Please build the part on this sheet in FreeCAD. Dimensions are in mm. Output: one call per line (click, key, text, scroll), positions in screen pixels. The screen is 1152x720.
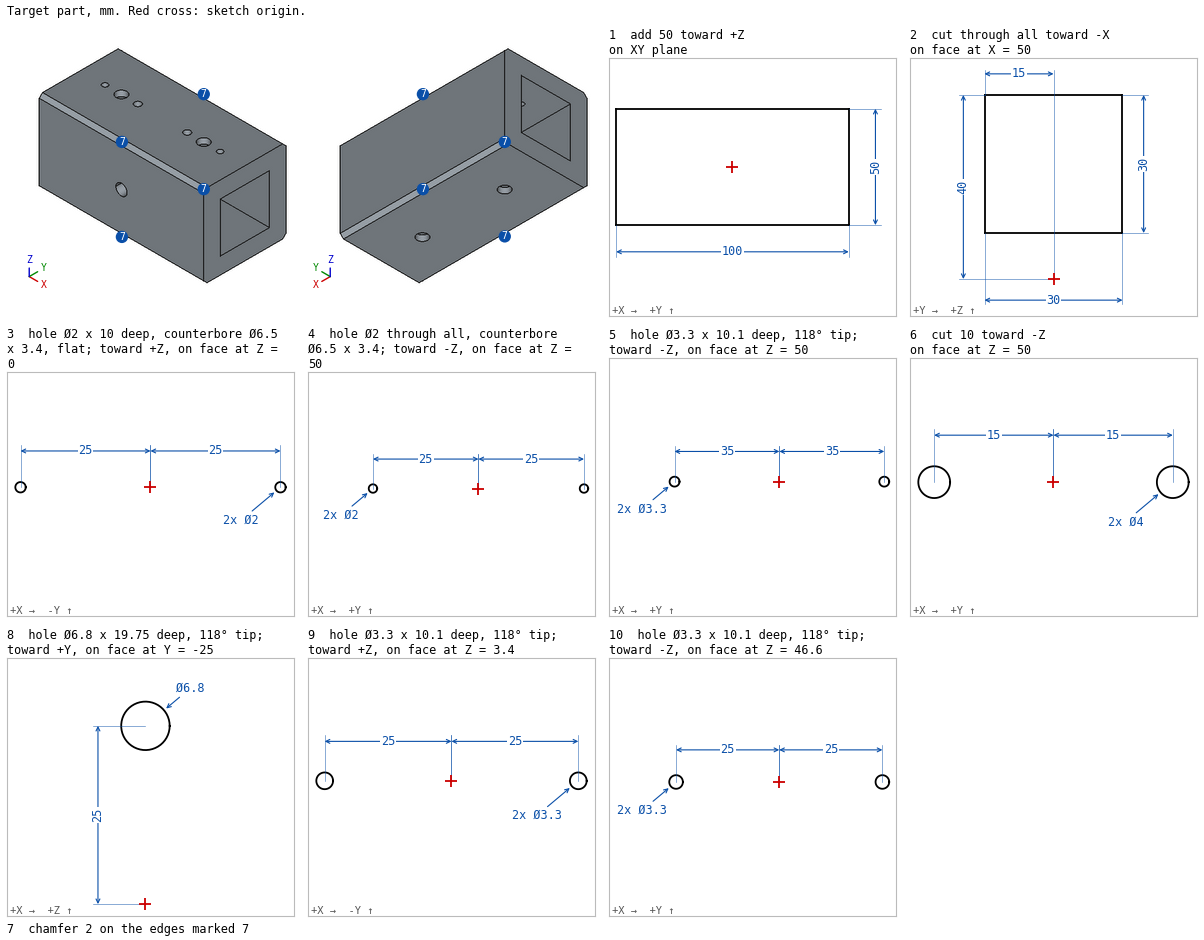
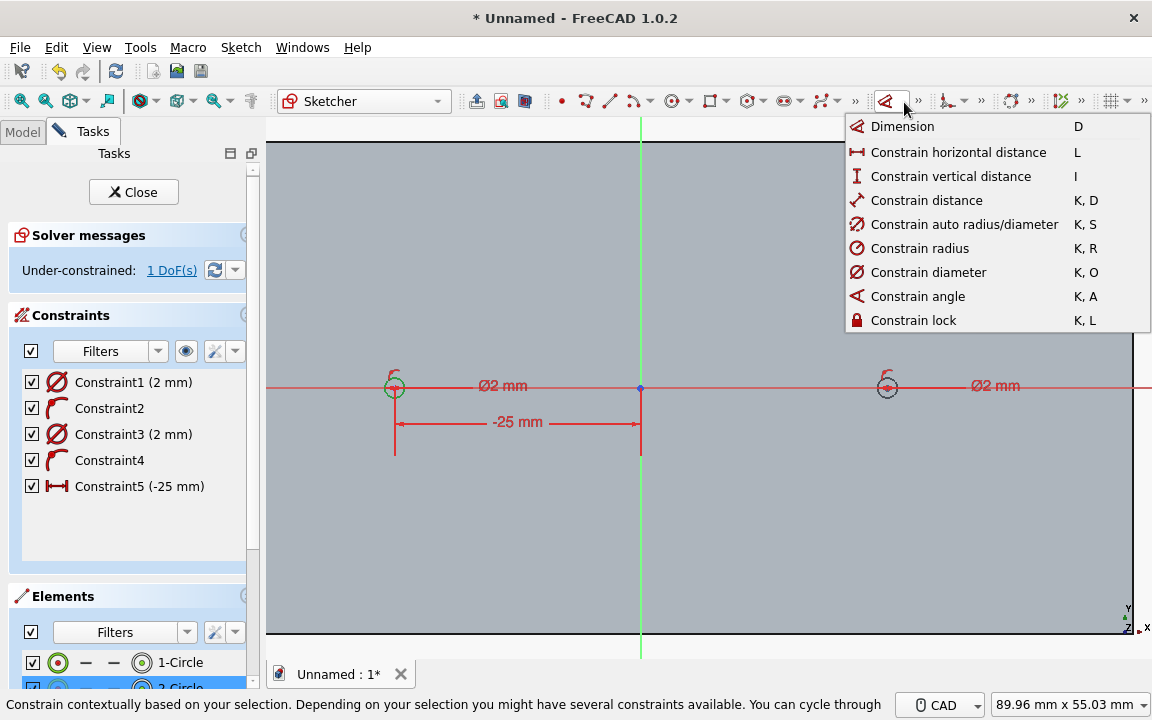
click(998, 152)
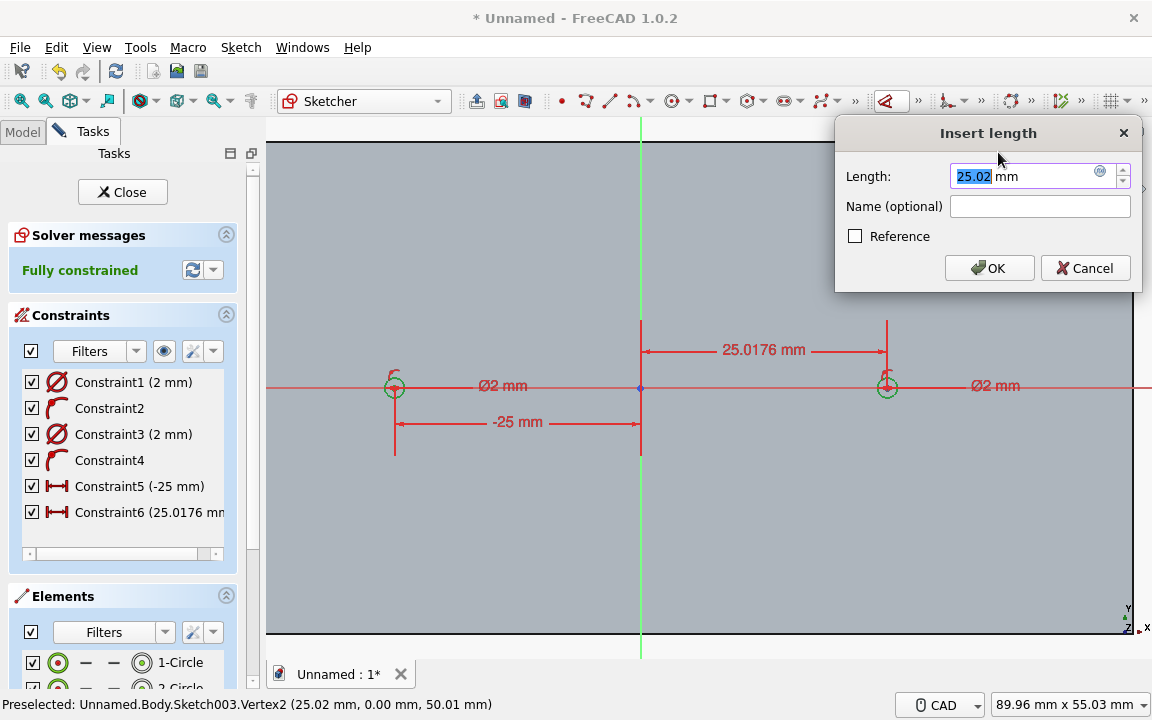
text(25)
key(Return)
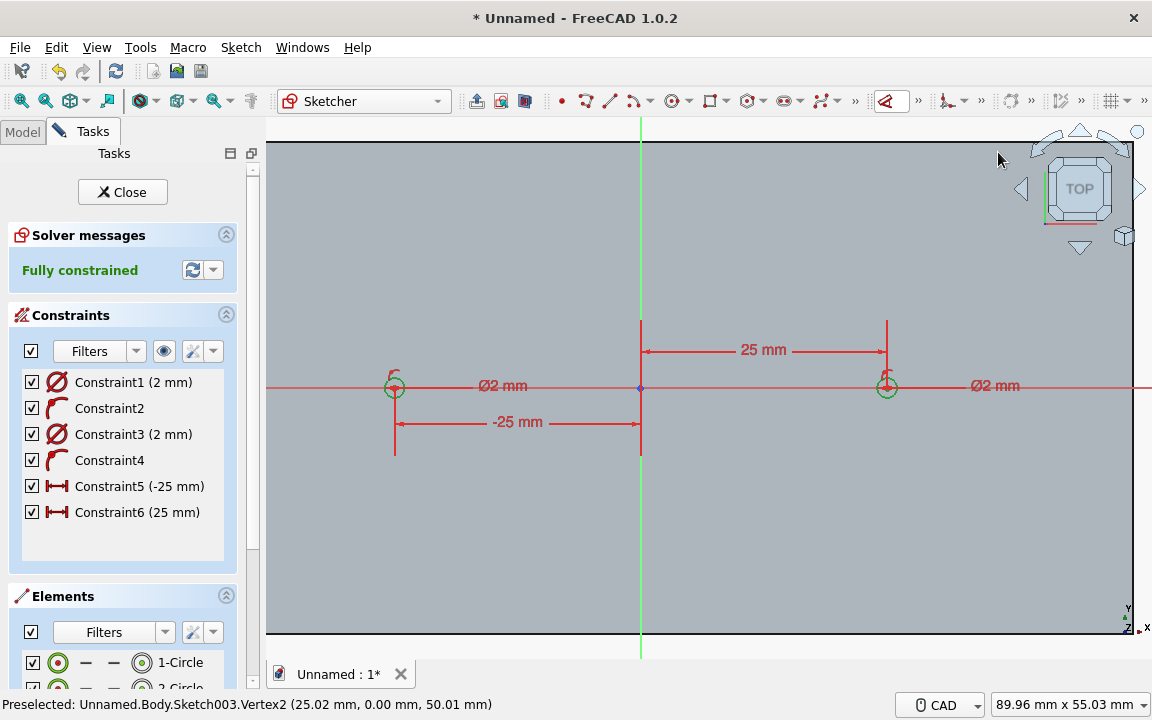
click(123, 192)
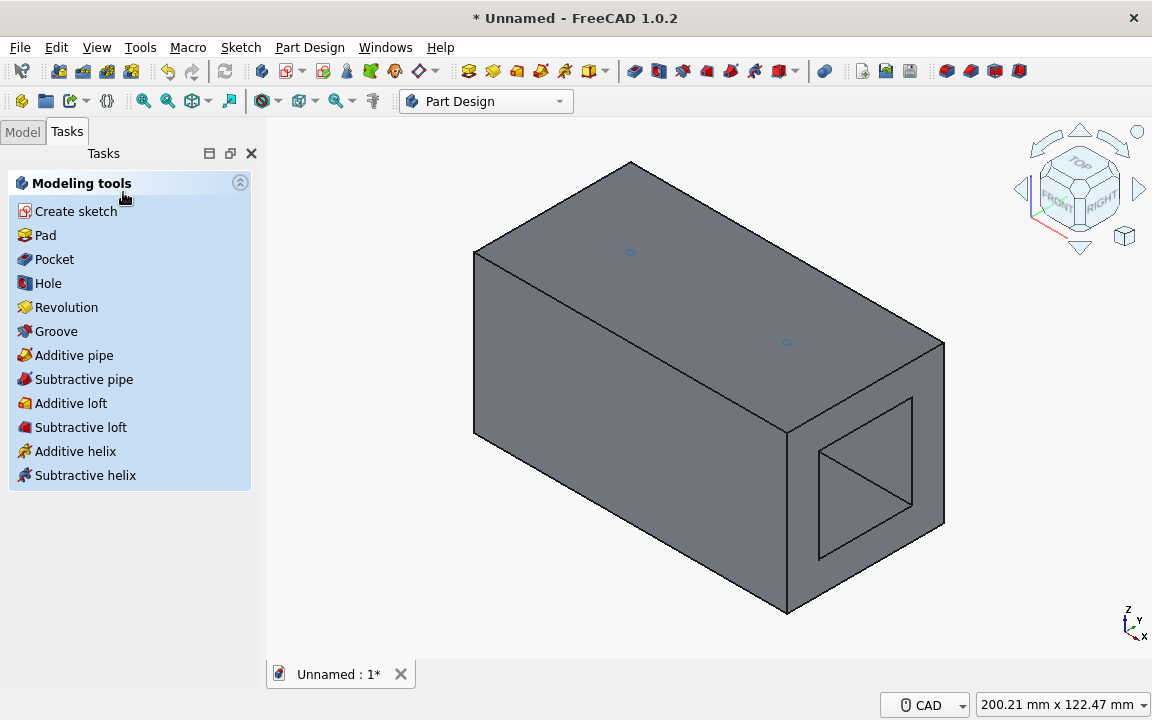
click(660, 72)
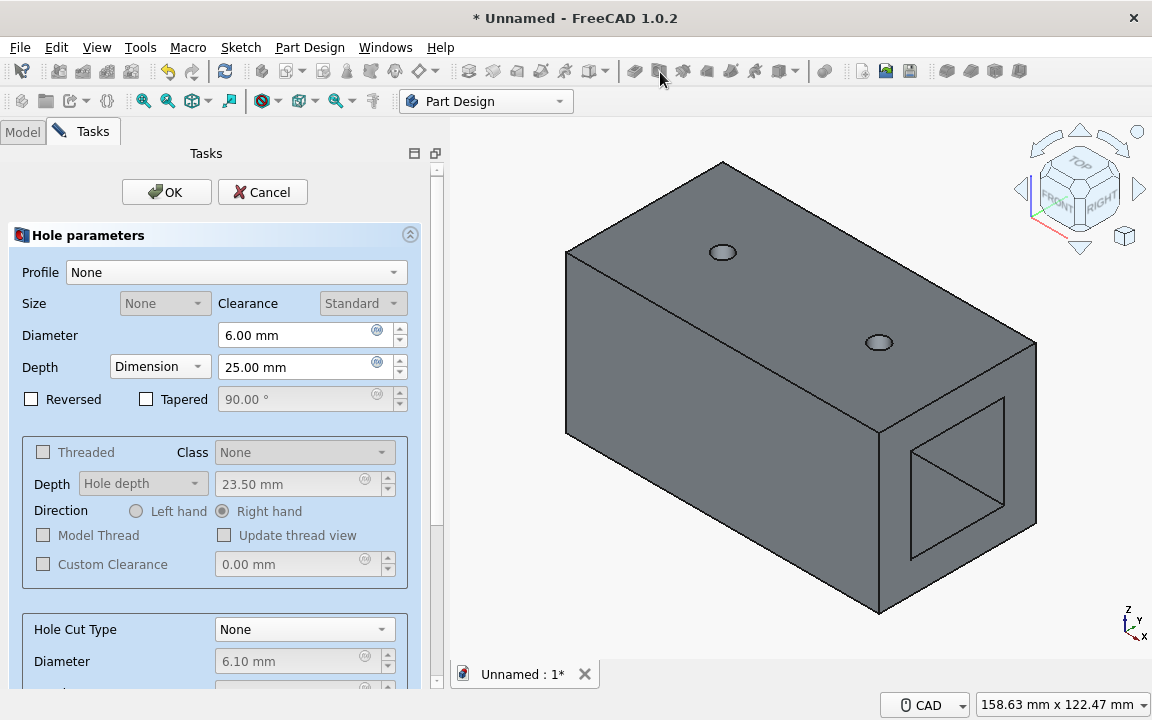
triple_click(305, 335)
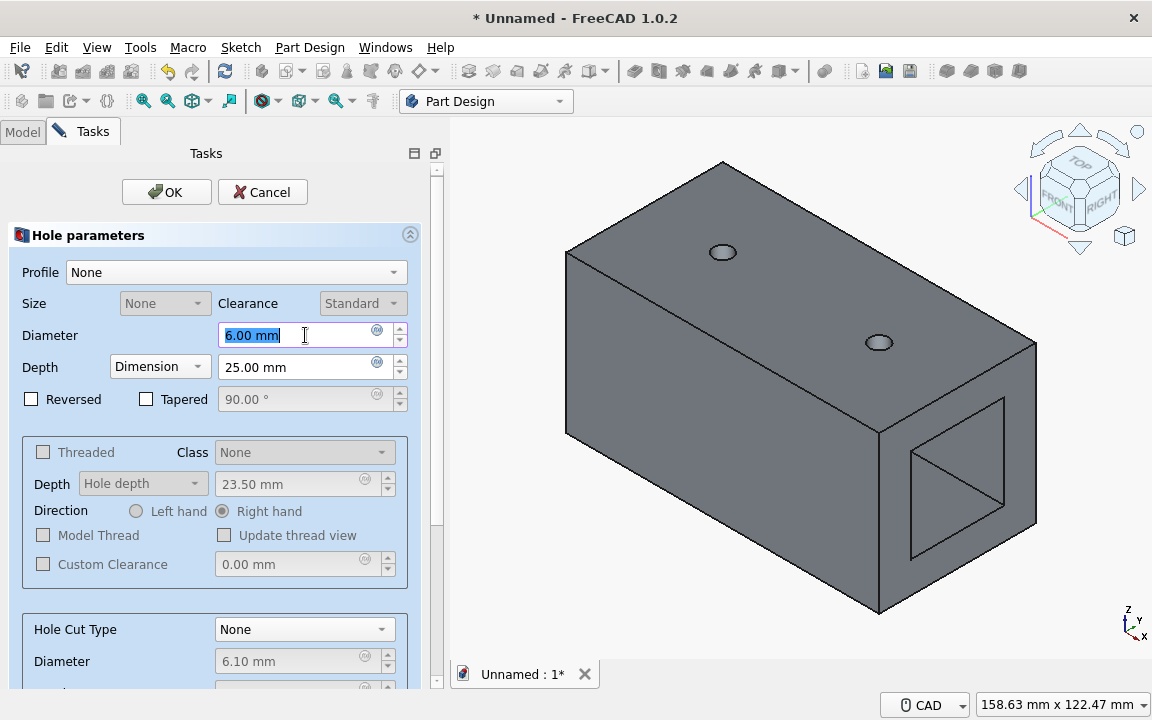
text(2)
key(Tab)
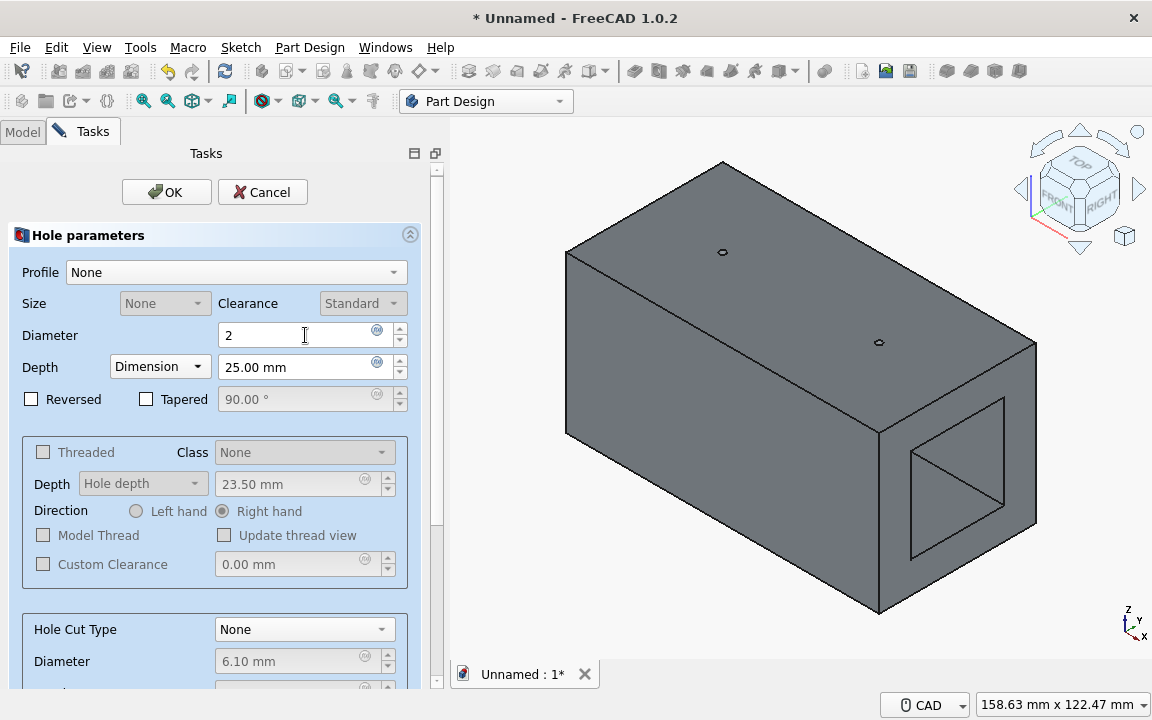
click(161, 366)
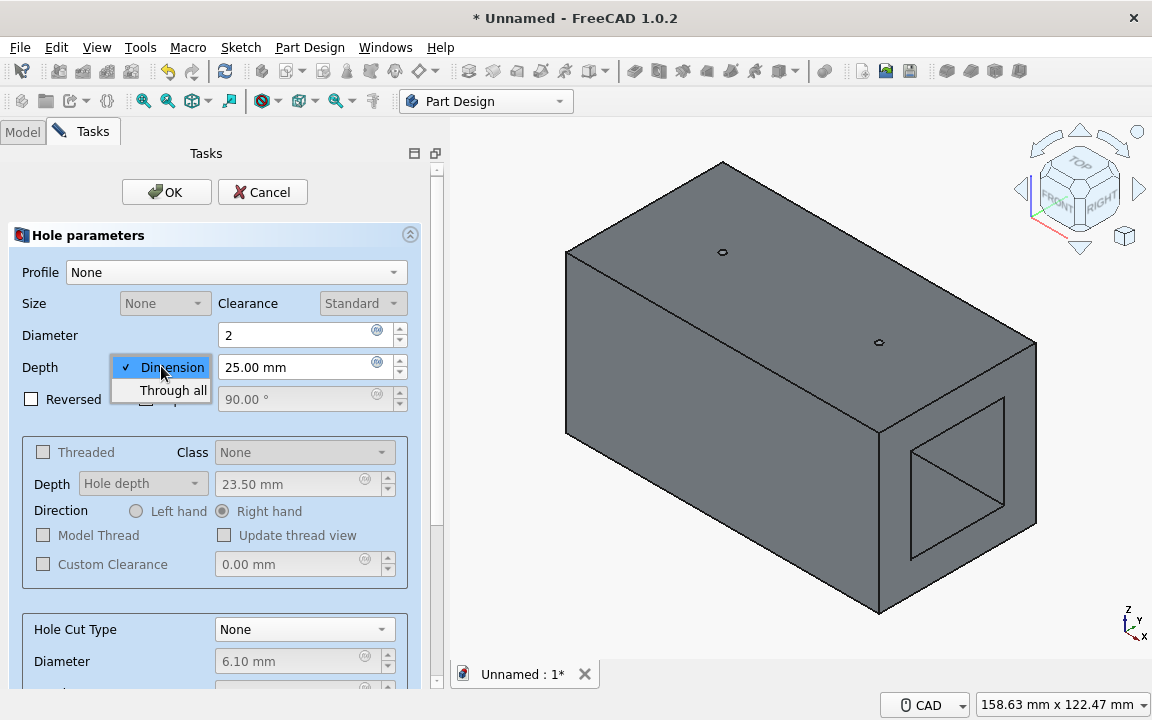
click(160, 390)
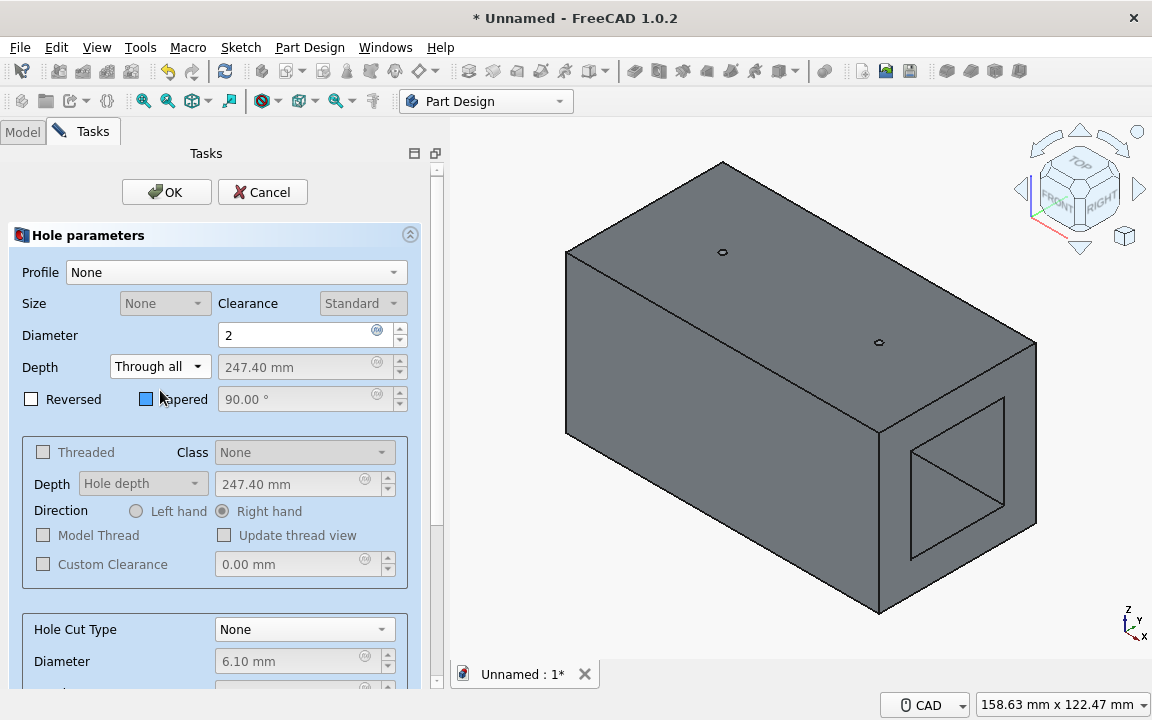
click(306, 630)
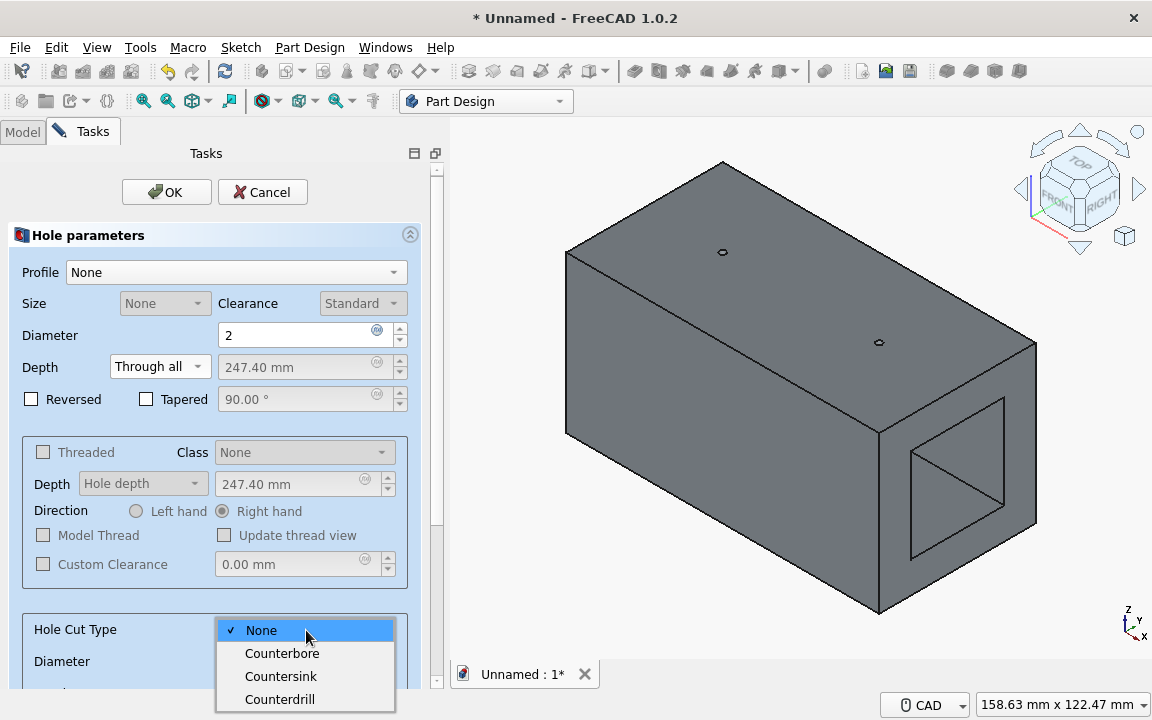
click(304, 654)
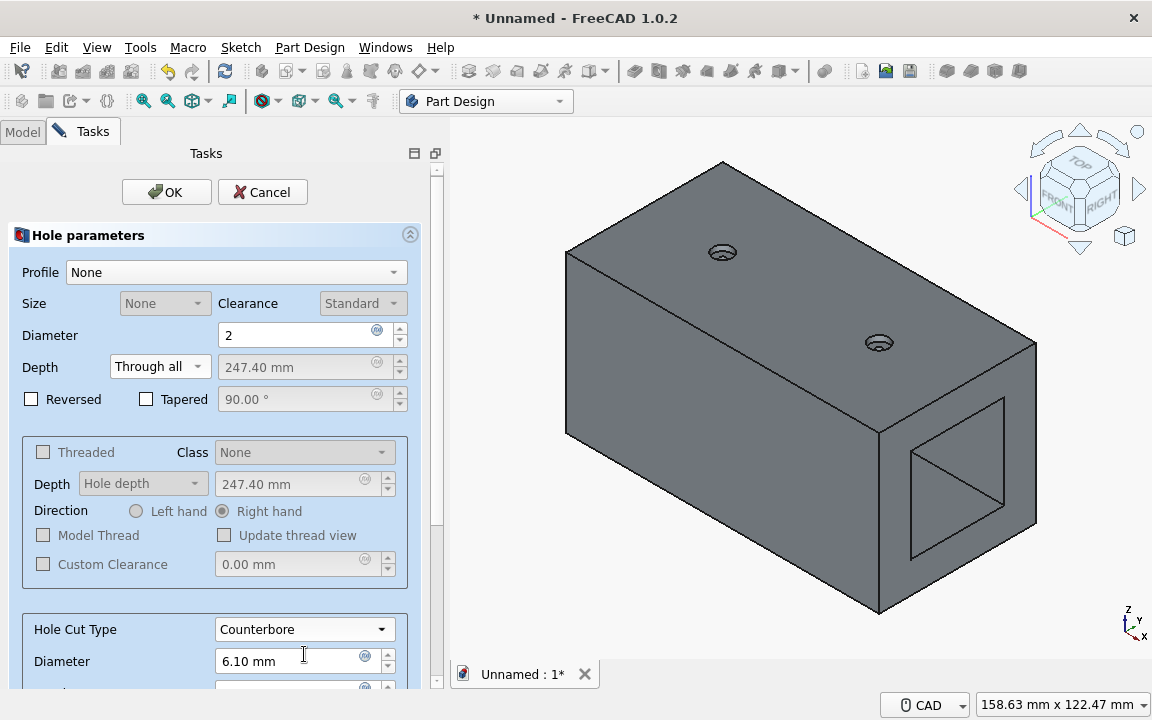
triple_click(298, 661)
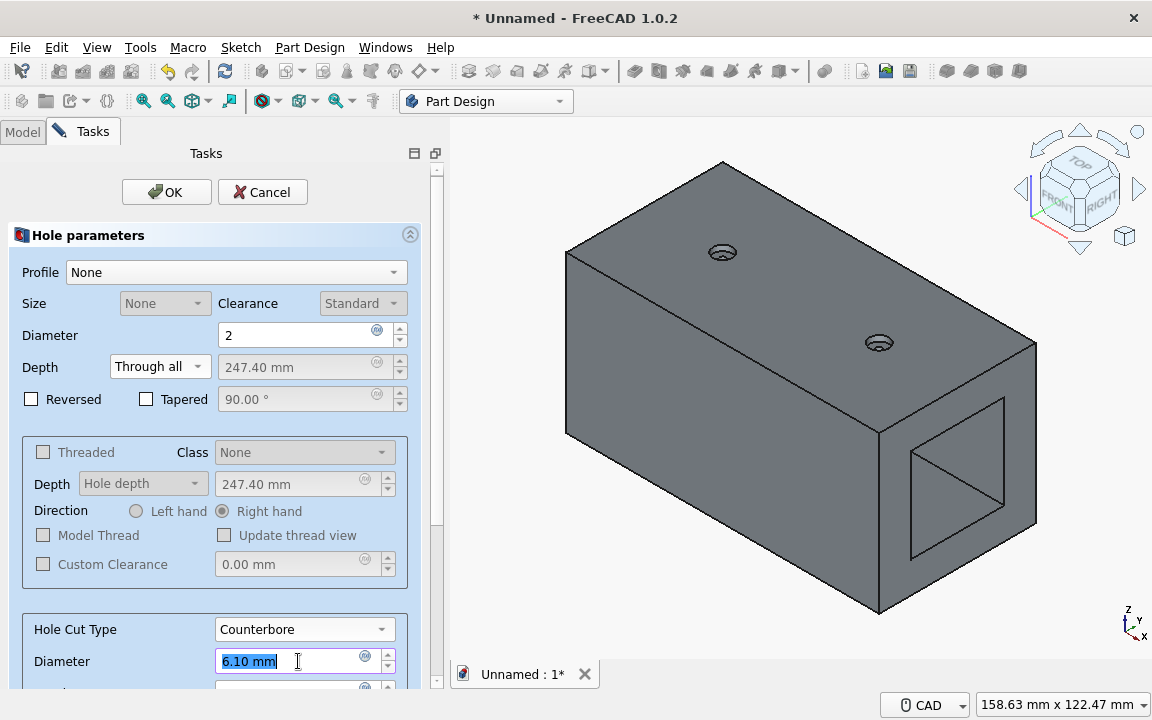
text(6.5)
key(Tab)